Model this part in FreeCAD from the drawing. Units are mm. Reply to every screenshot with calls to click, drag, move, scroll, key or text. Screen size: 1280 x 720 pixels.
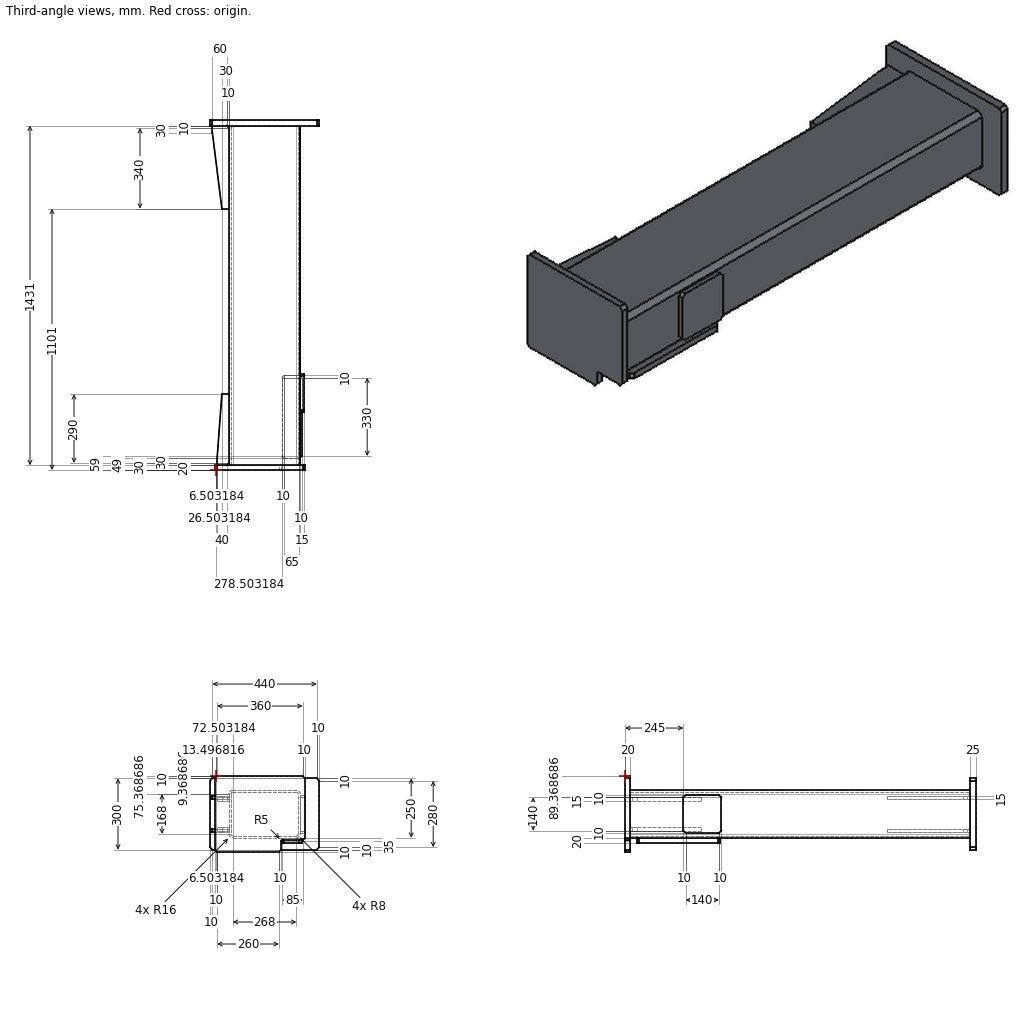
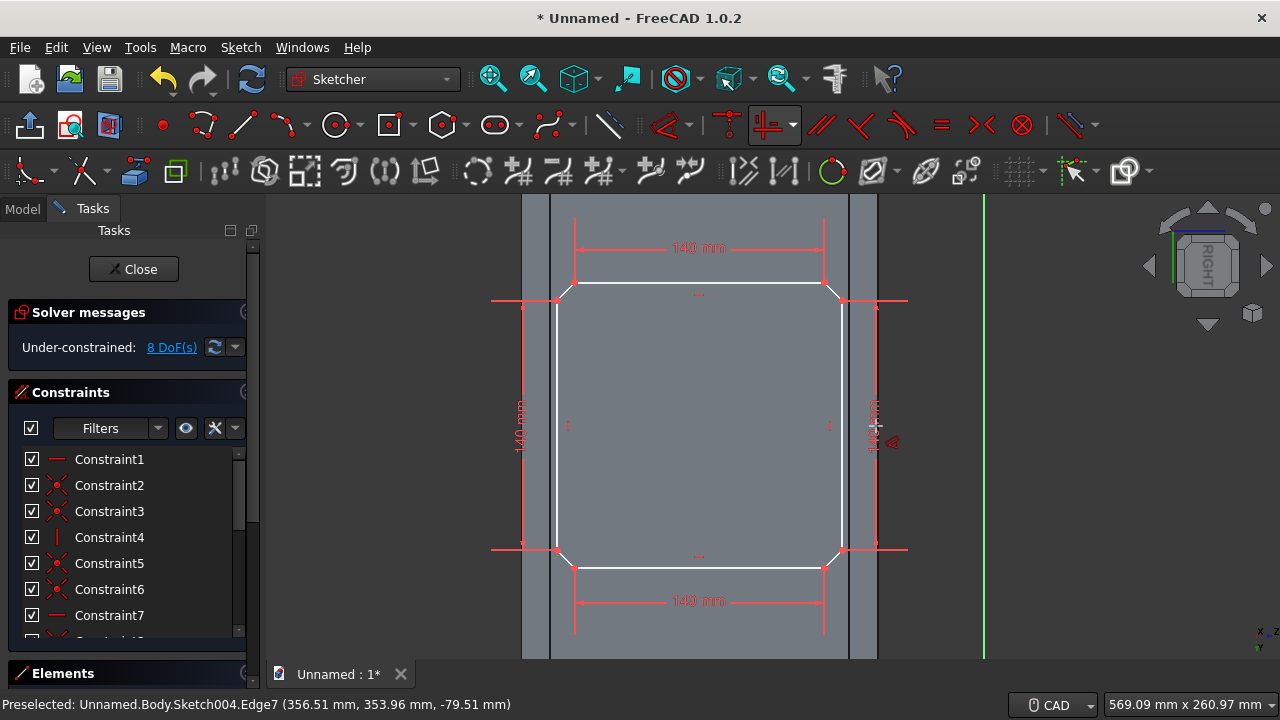
scroll(568, 290, up, 5)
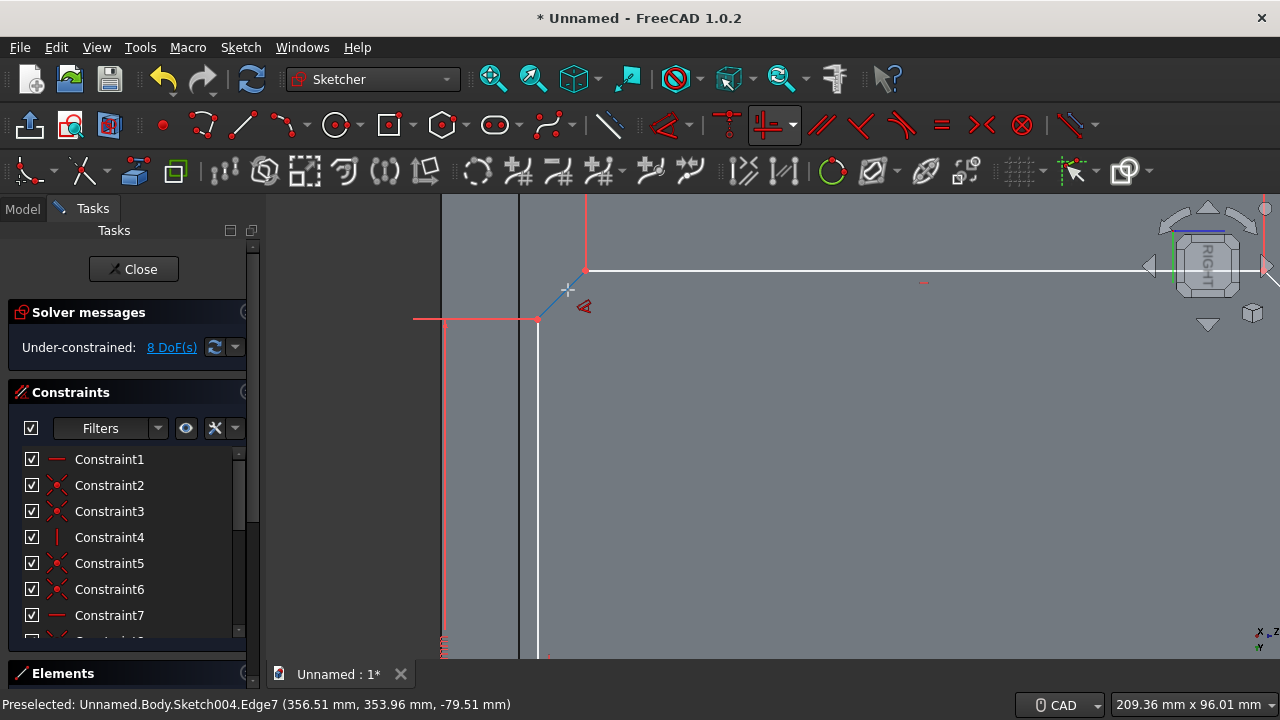
click(566, 290)
click(562, 237)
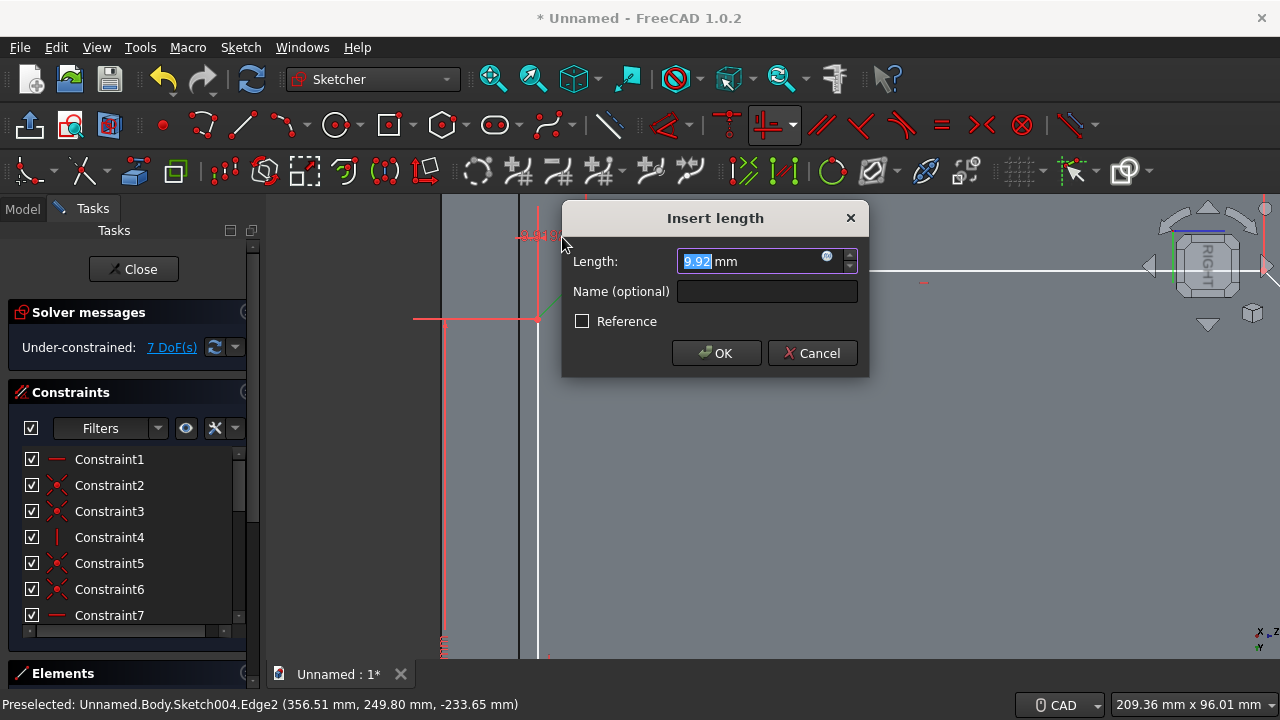
text(10)
key(Return)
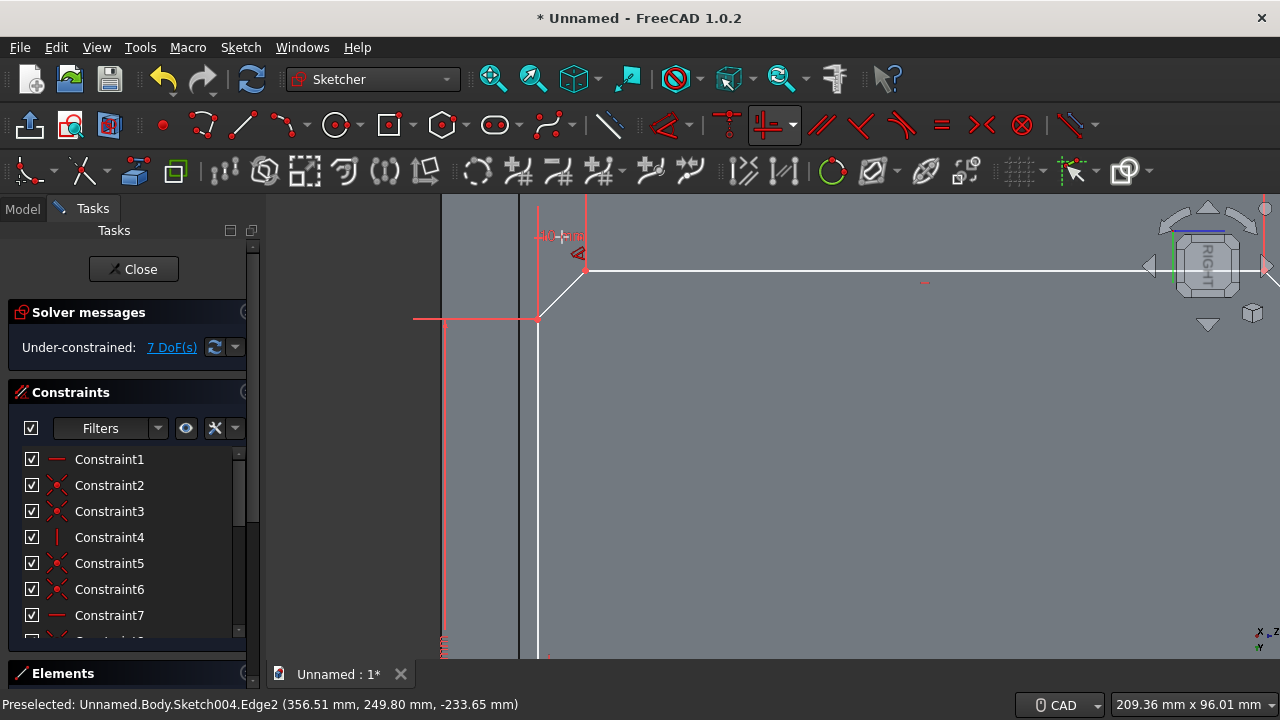
click(571, 285)
click(504, 295)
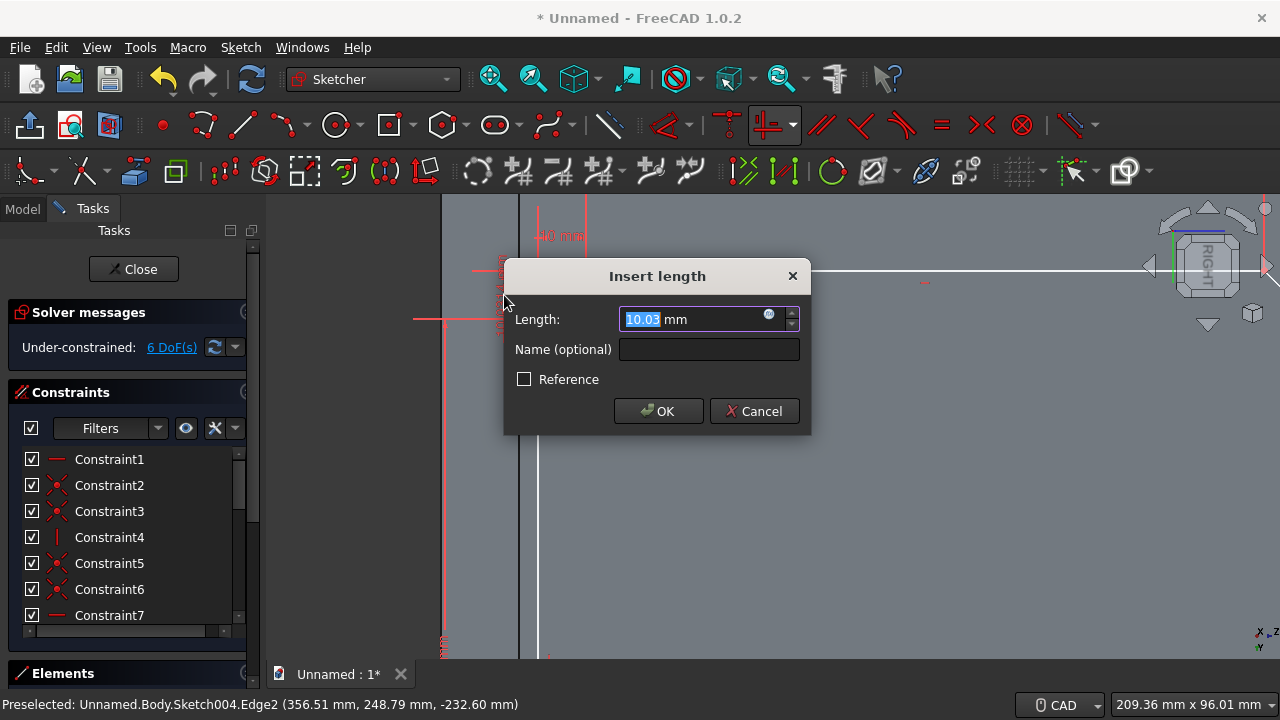
text(10)
key(Return)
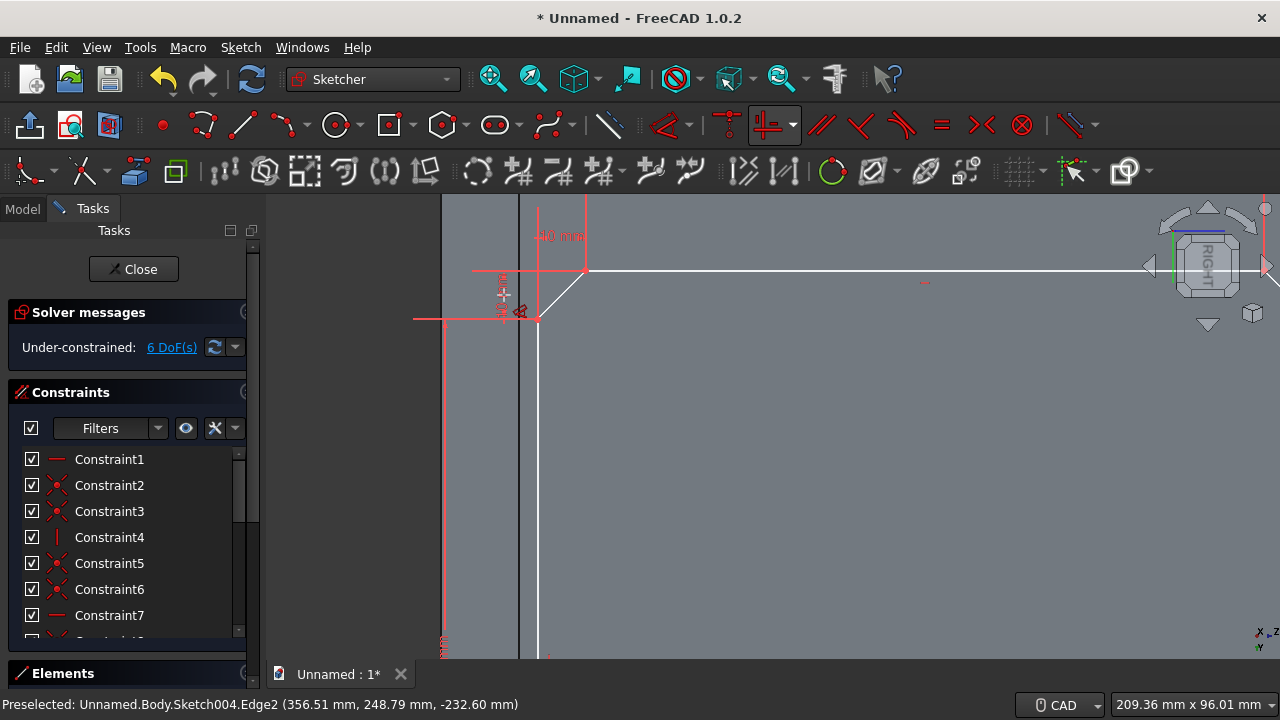
scroll(576, 294, down, 5)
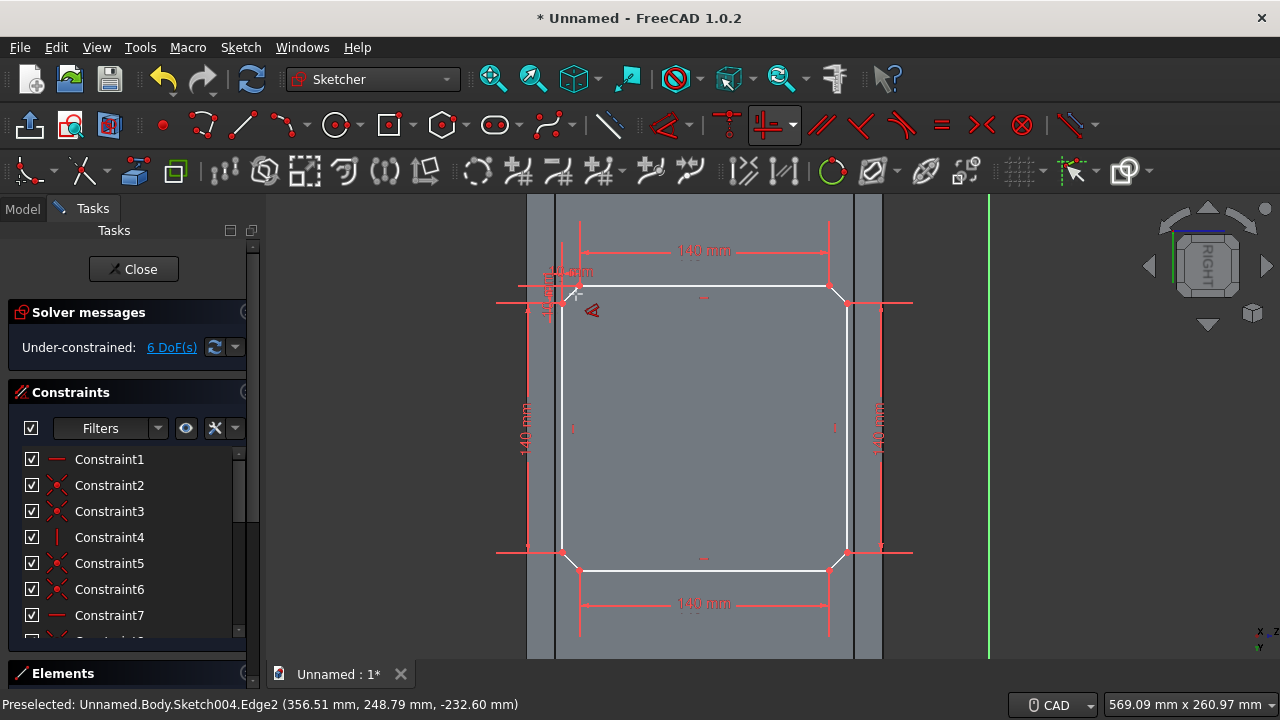
scroll(567, 558, up, 5)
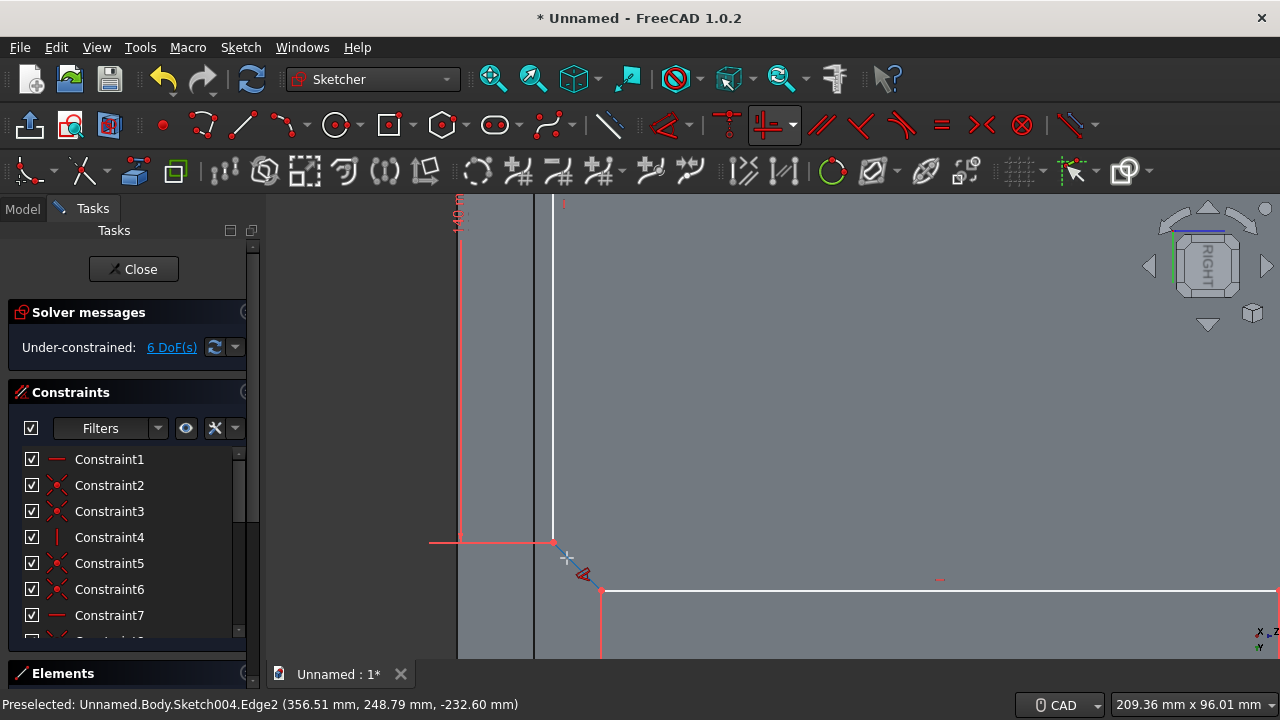
click(567, 557)
click(577, 625)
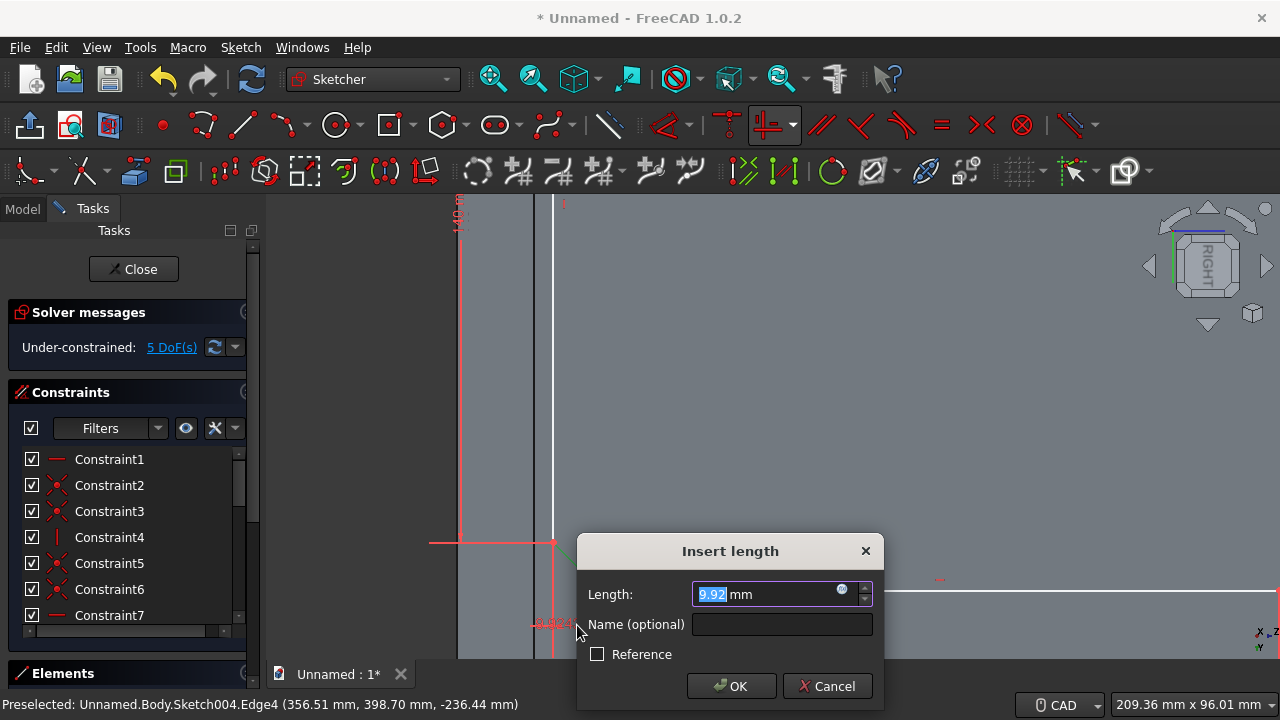
text(10)
key(Return)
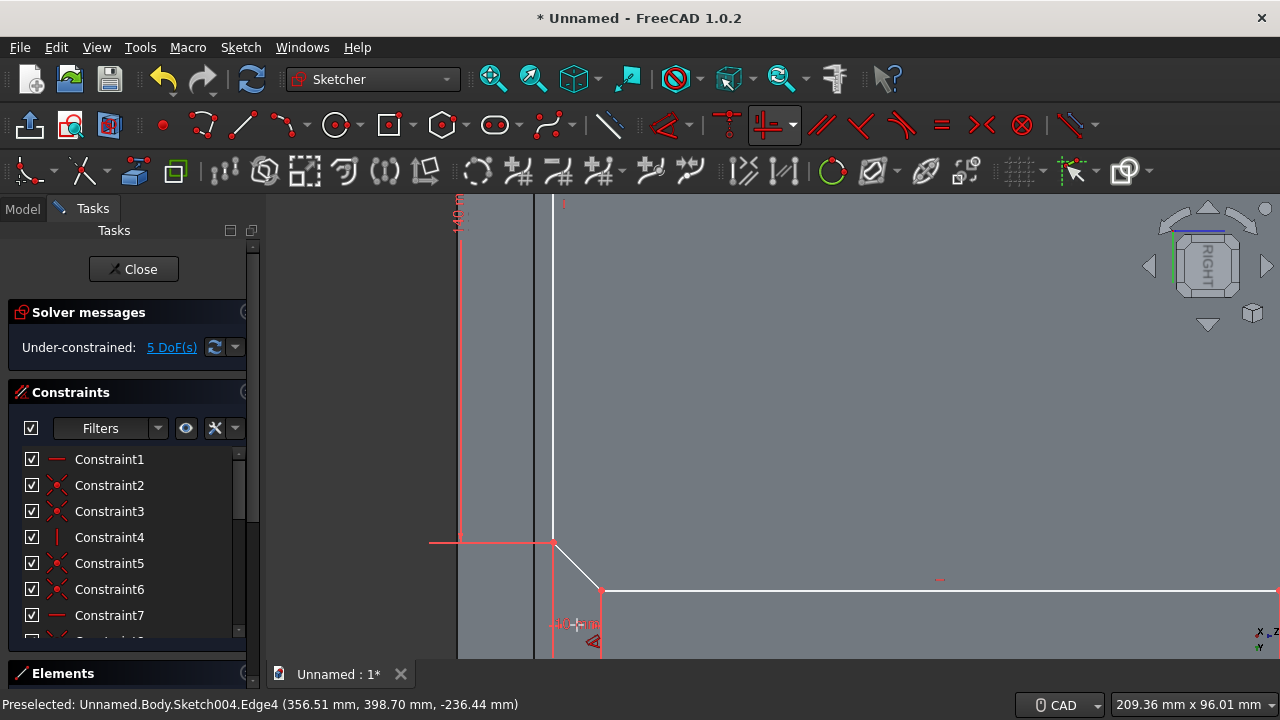
click(568, 557)
click(519, 567)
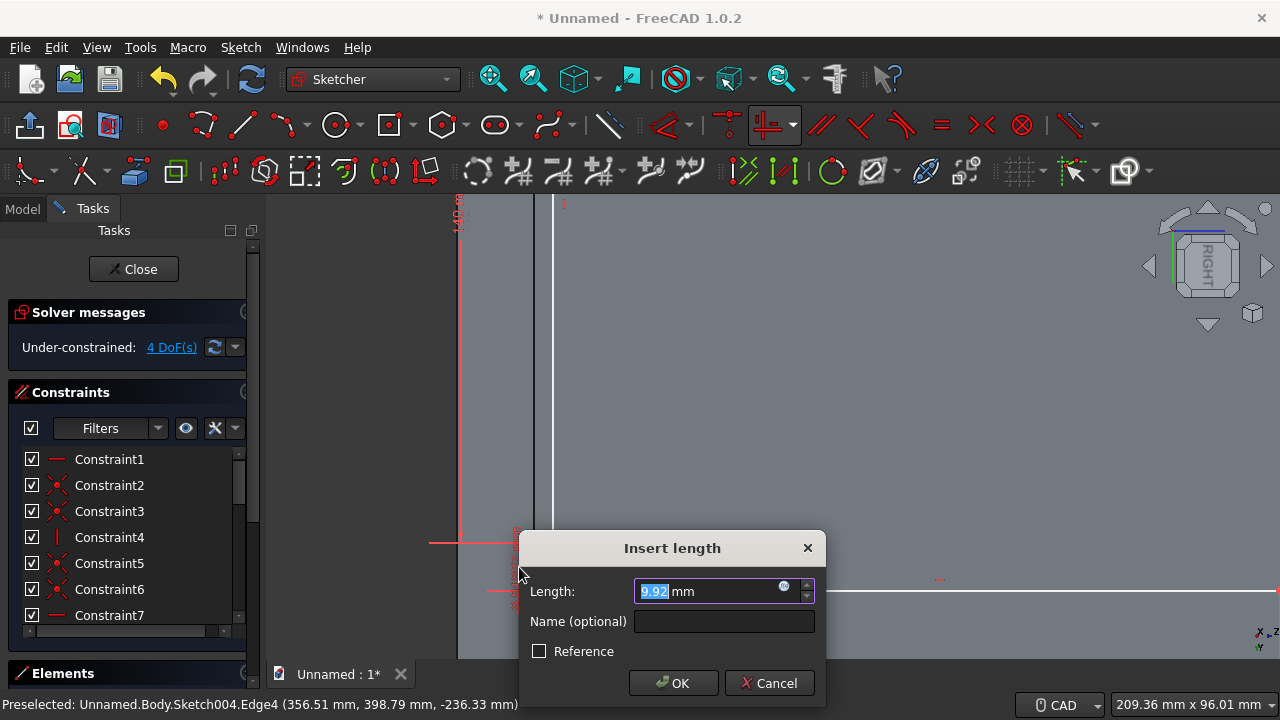
text(10)
key(Return)